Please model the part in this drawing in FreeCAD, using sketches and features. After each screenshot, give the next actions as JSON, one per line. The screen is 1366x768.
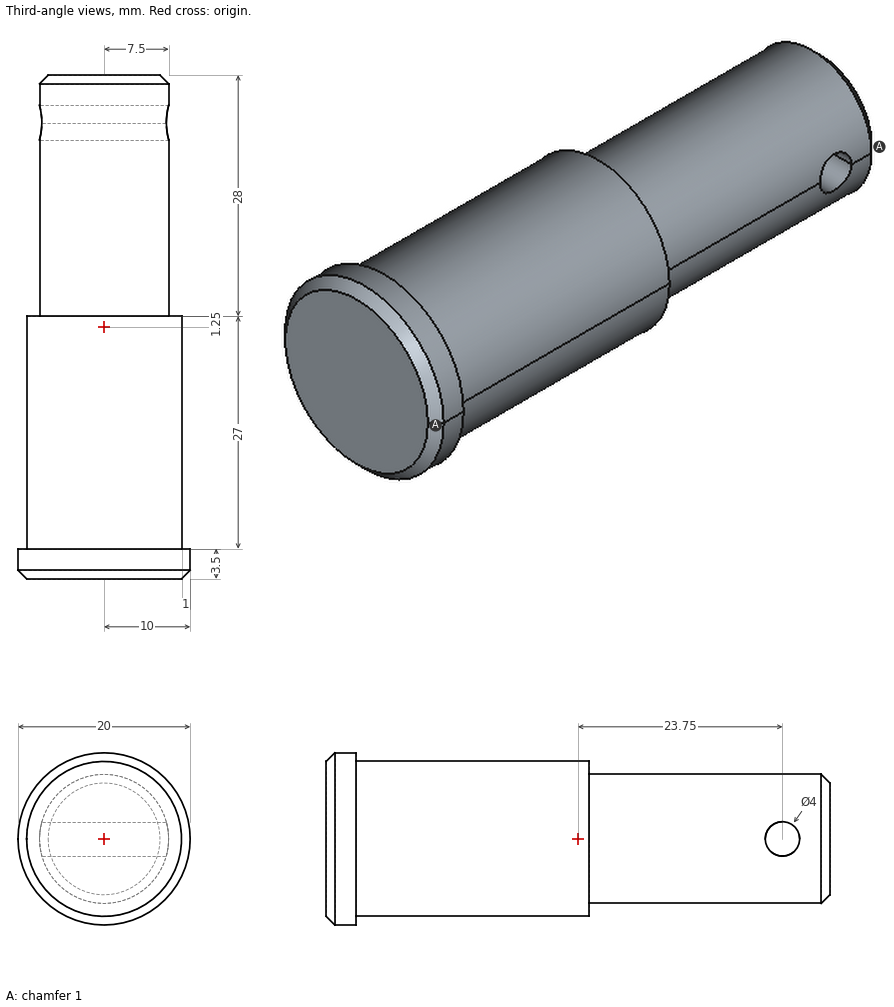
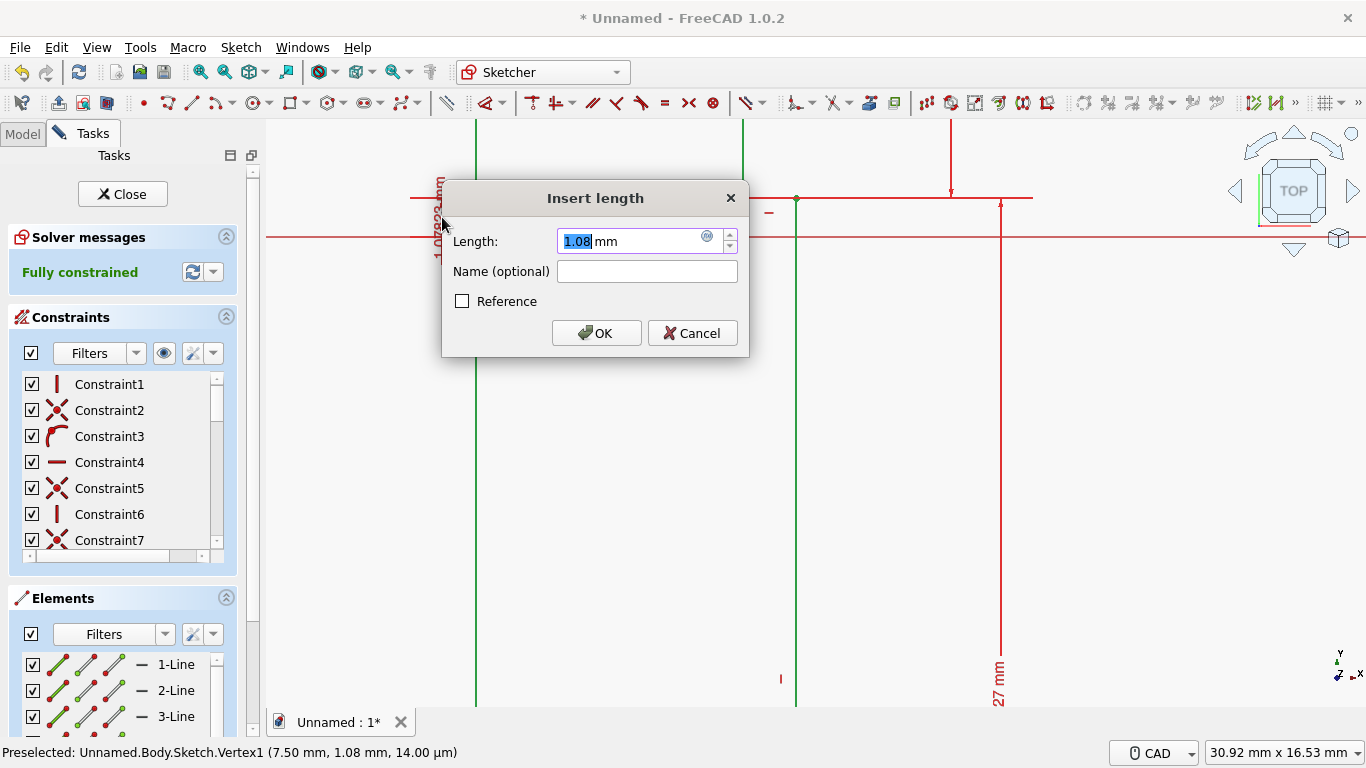
{"action": "type", "text": "1.25"}
{"action": "key", "text": "Return"}
{"action": "key", "text": "Escape"}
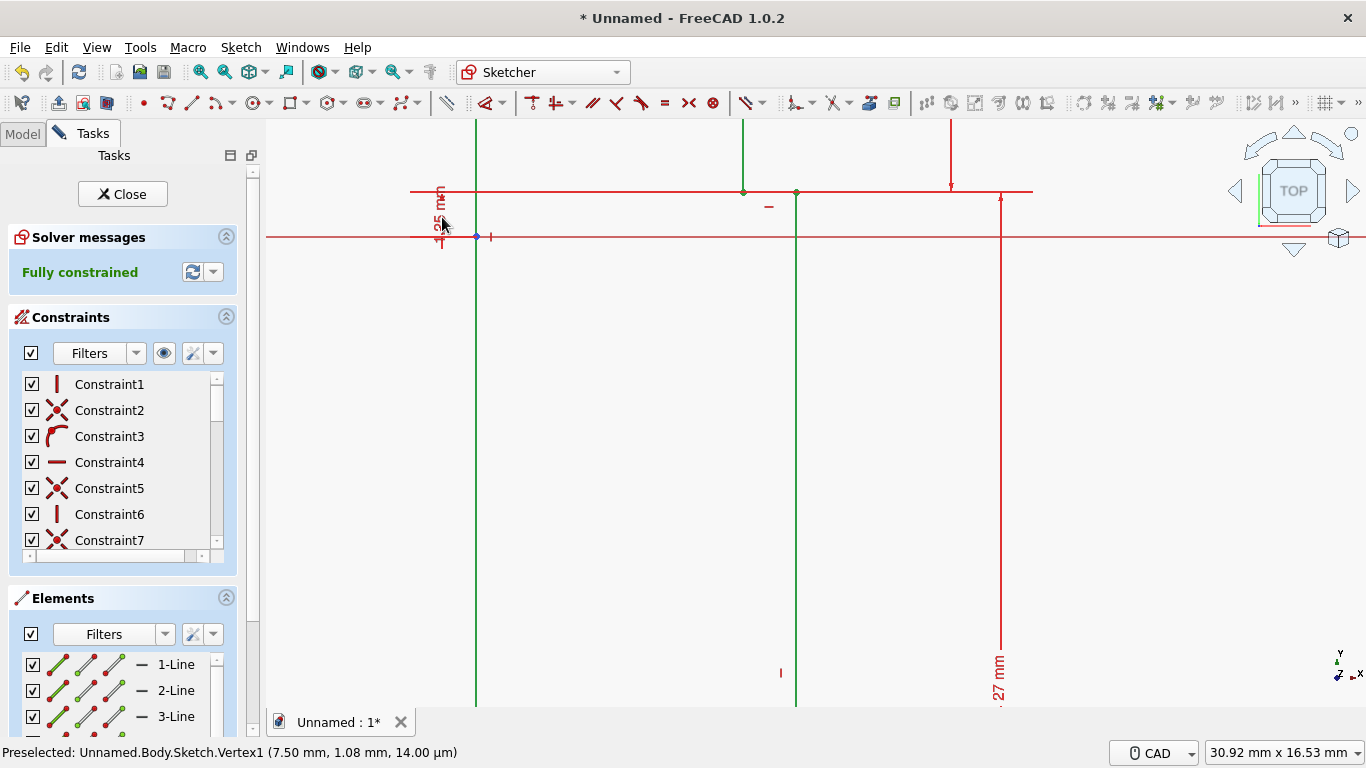
{"action": "left_click", "coordinate": [123, 194]}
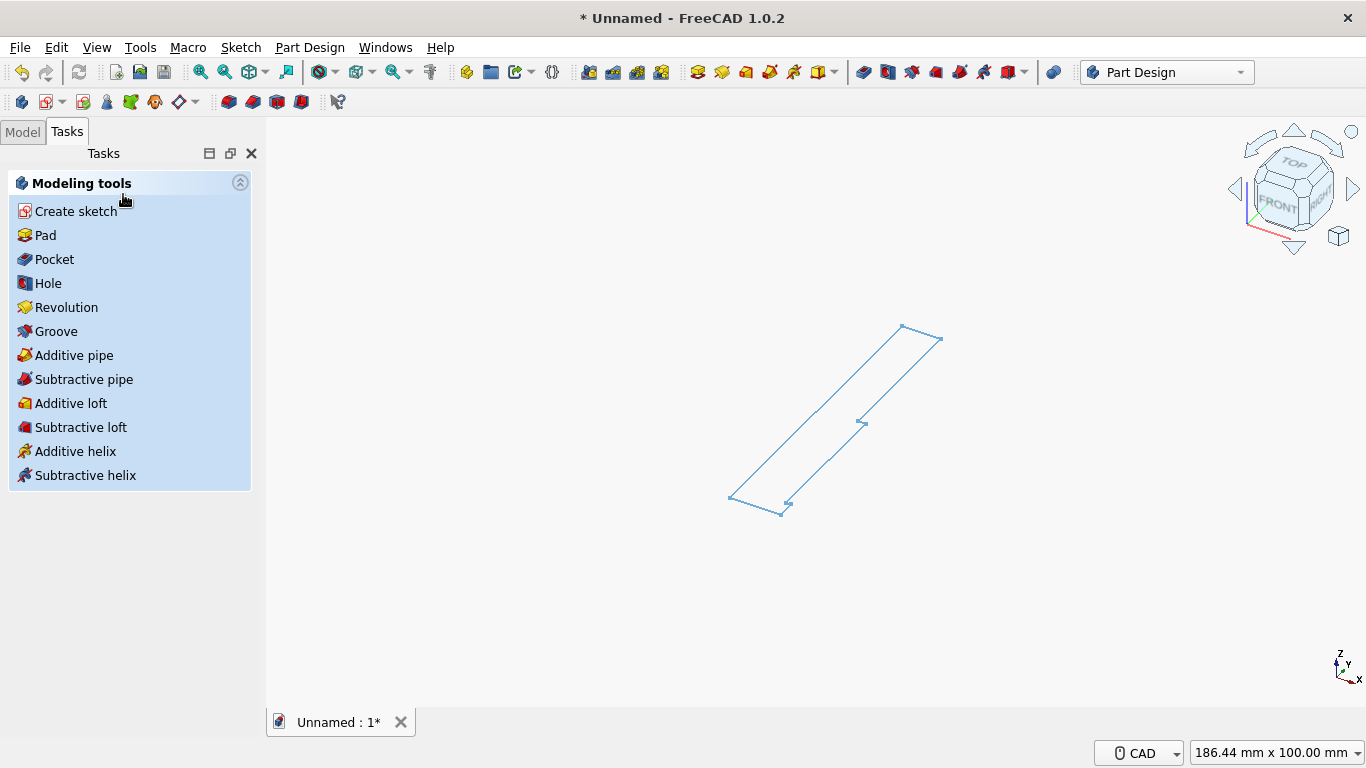
{"action": "left_click", "coordinate": [722, 72]}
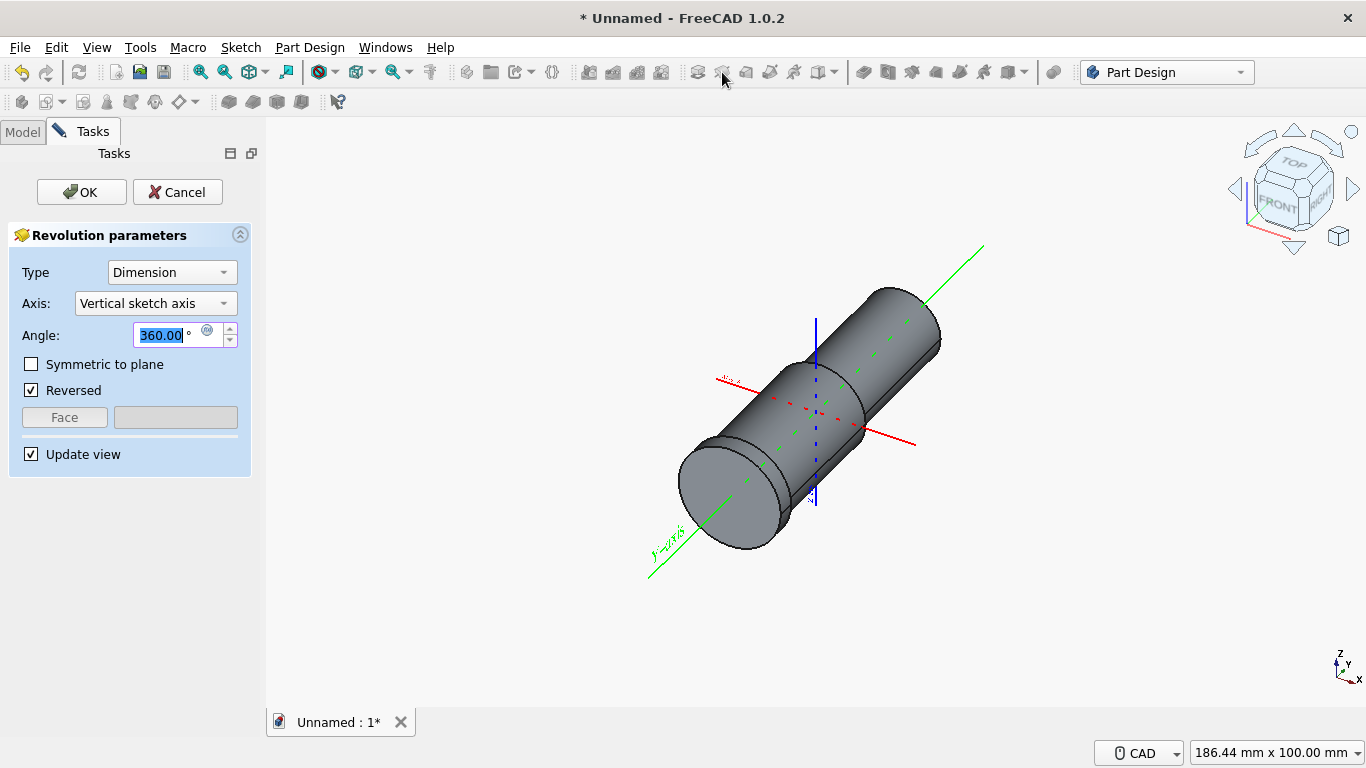
{"action": "left_click", "coordinate": [82, 192]}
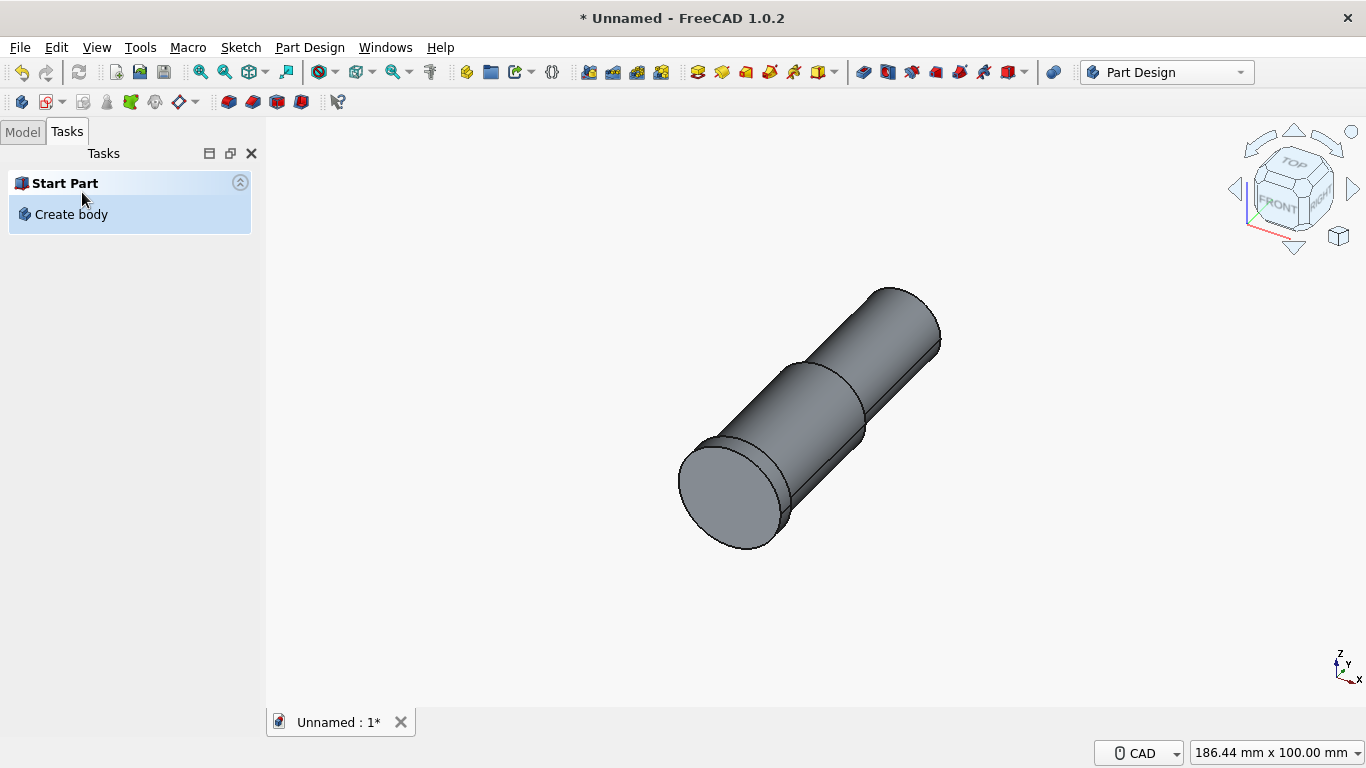
{"action": "left_click", "coordinate": [46, 102]}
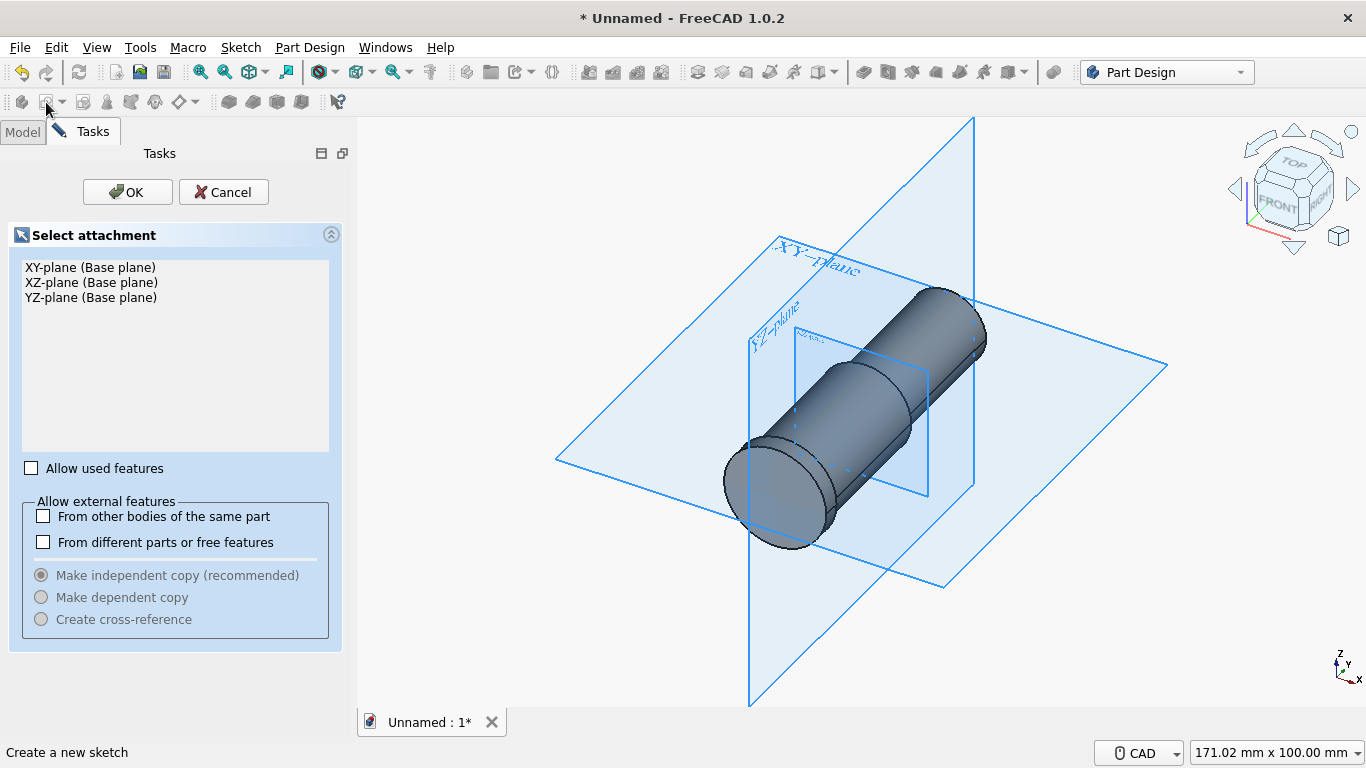
{"action": "left_click", "coordinate": [82, 298]}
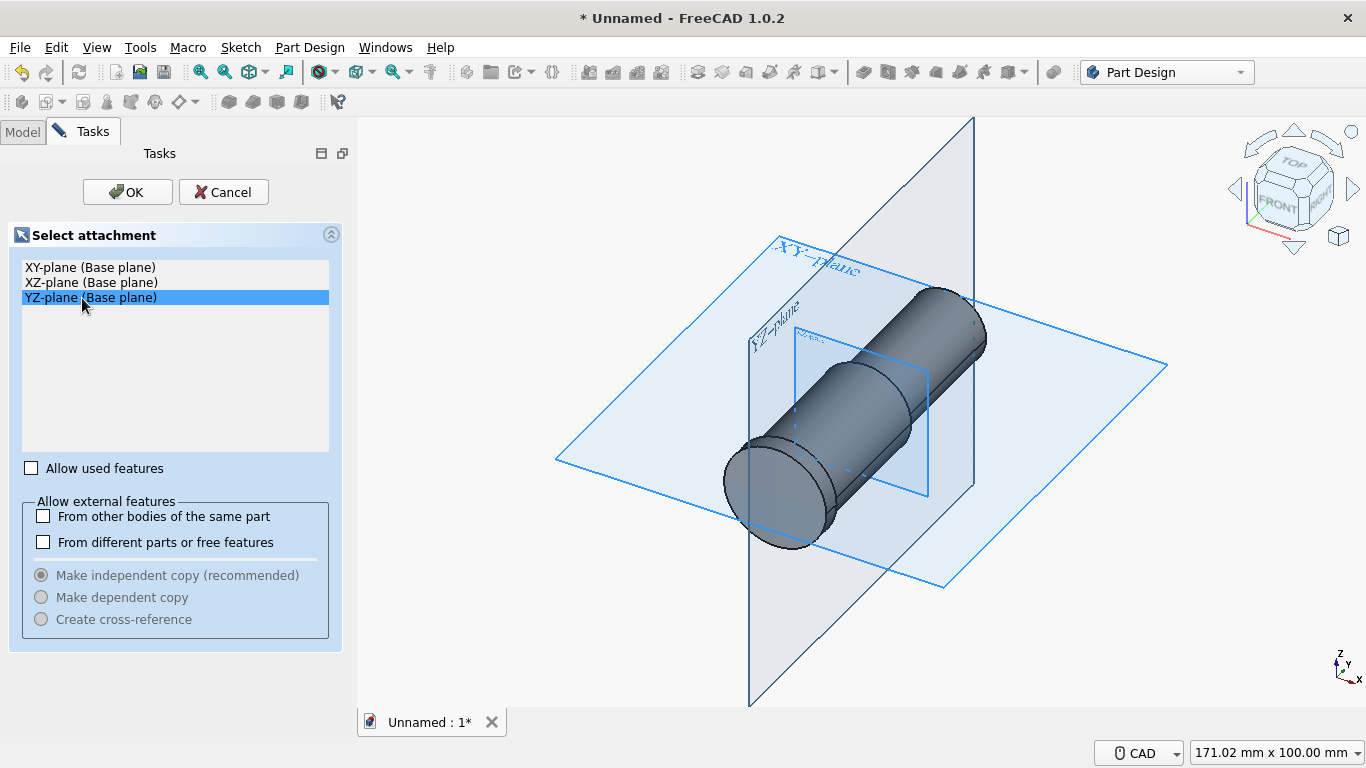
{"action": "left_click", "coordinate": [128, 192]}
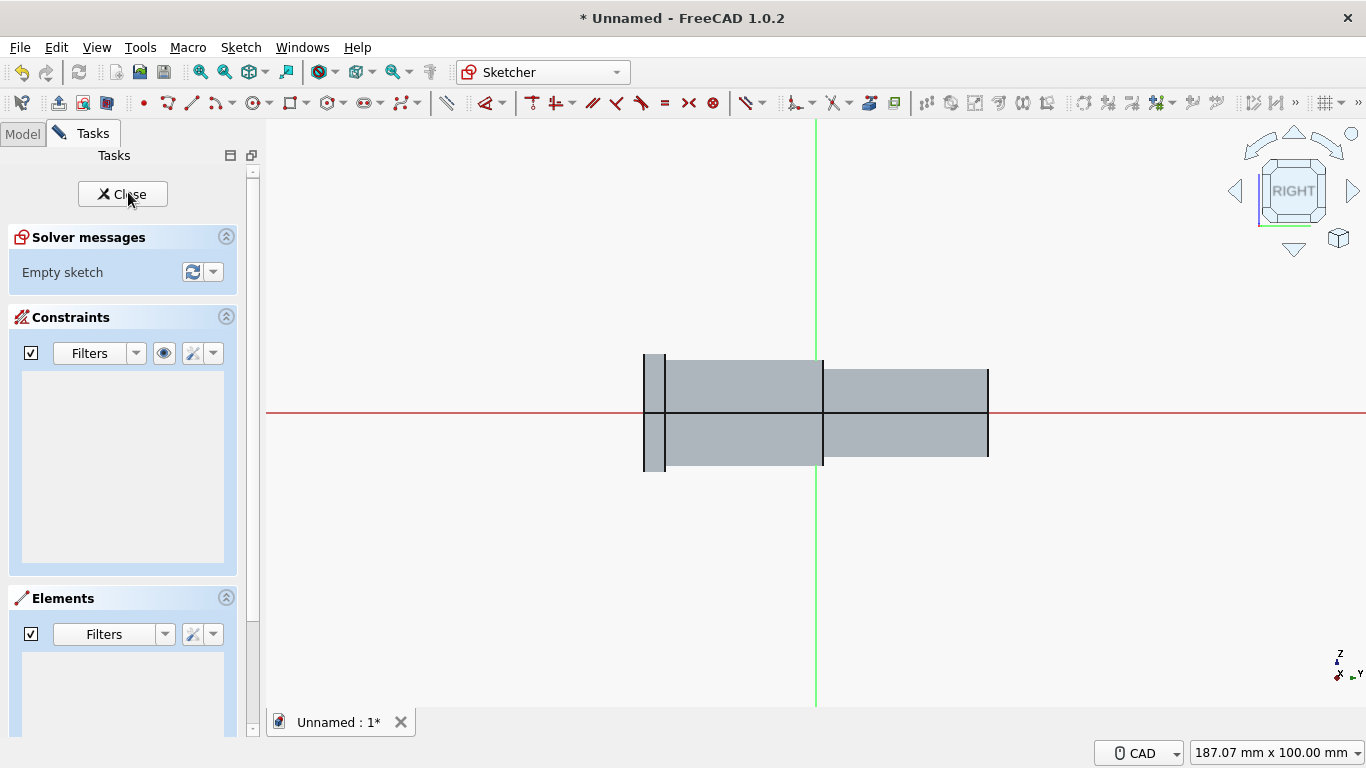
{"action": "left_click", "coordinate": [108, 104]}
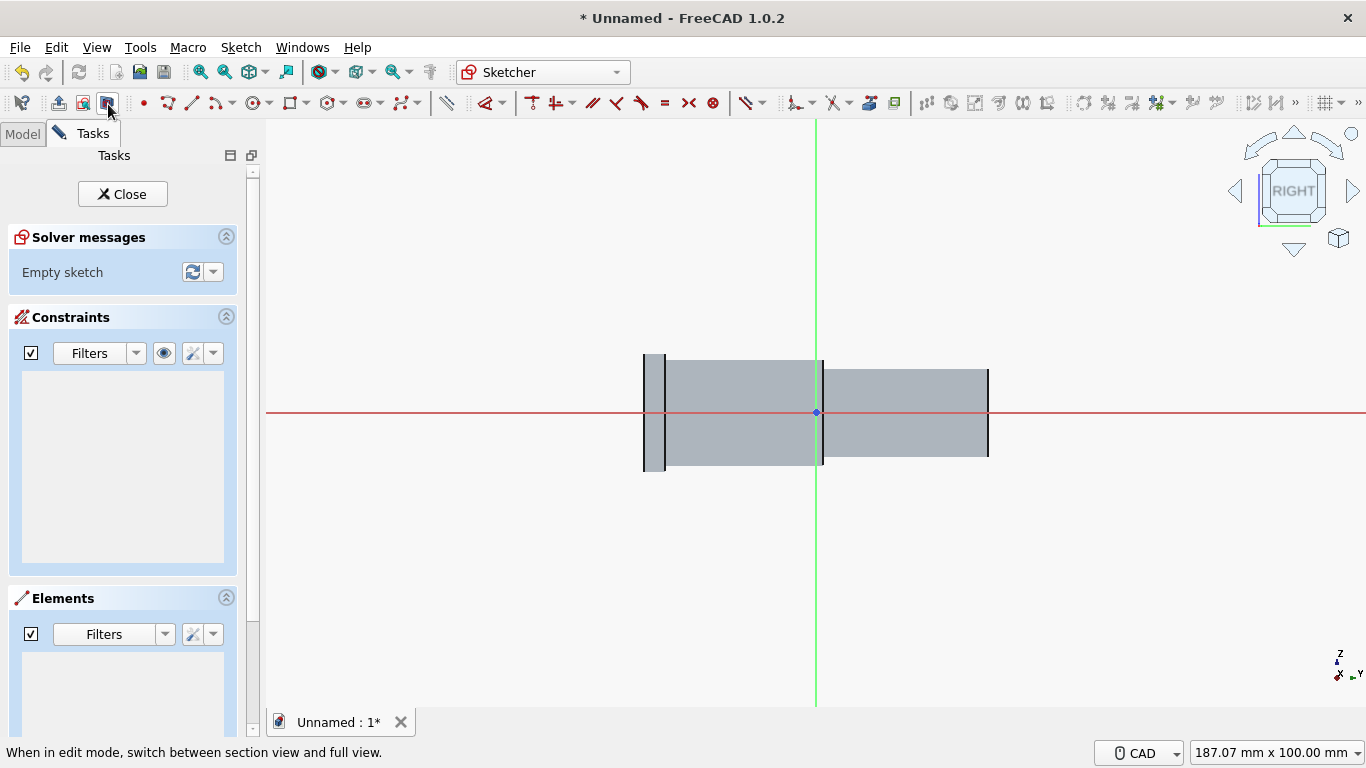
{"action": "scroll", "coordinate": [969, 413], "scroll_direction": "up", "scroll_amount": 14}